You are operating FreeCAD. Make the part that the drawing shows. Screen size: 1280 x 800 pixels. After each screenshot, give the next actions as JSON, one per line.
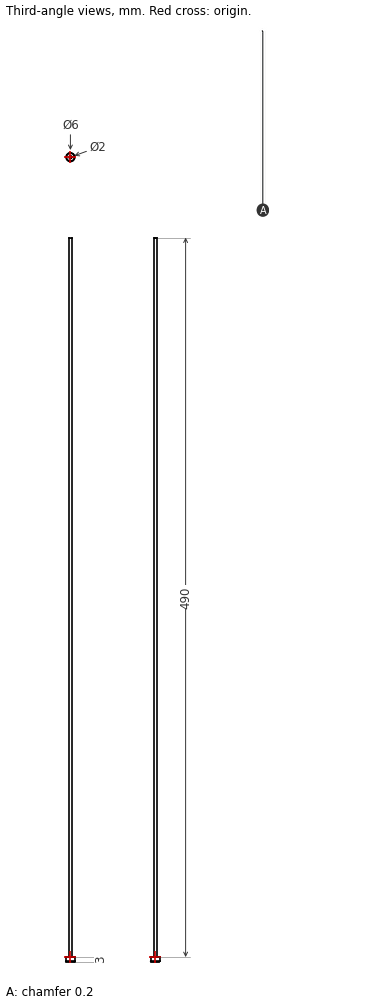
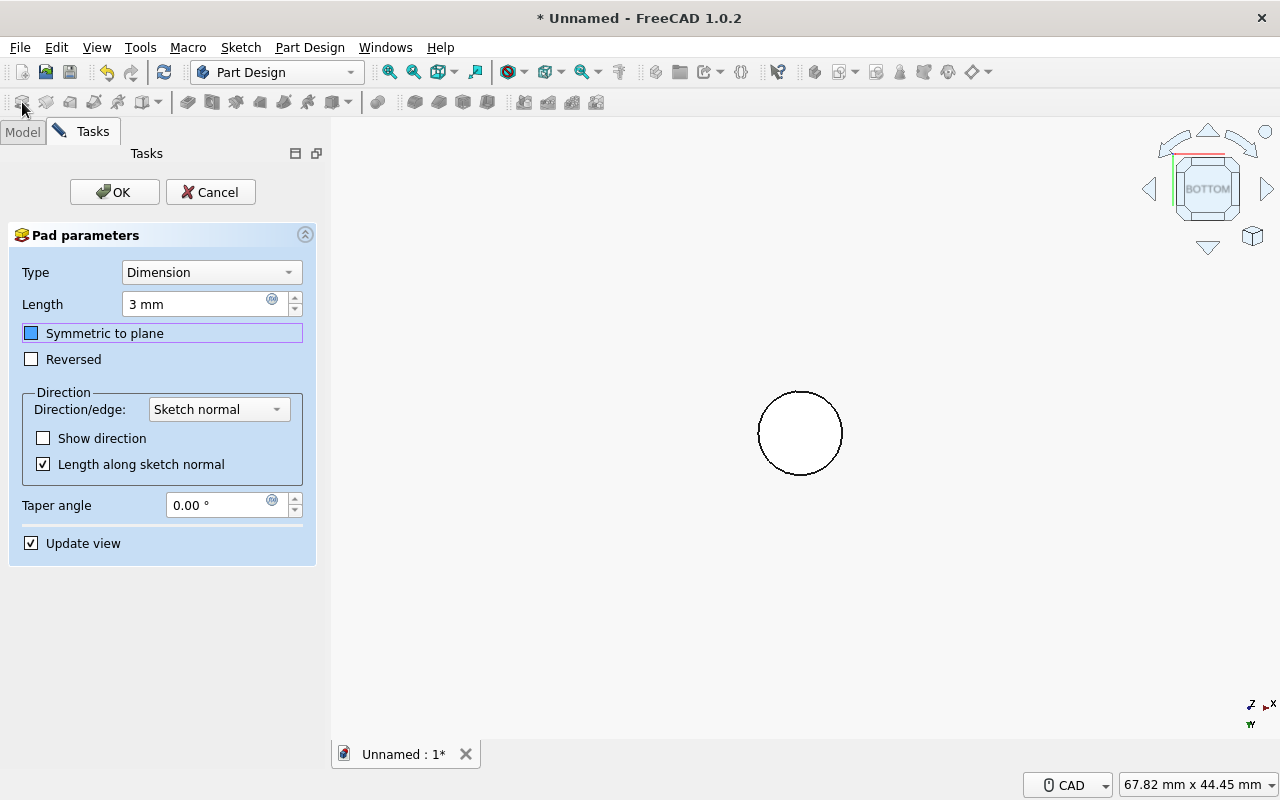
{"action": "left_click", "coordinate": [115, 192]}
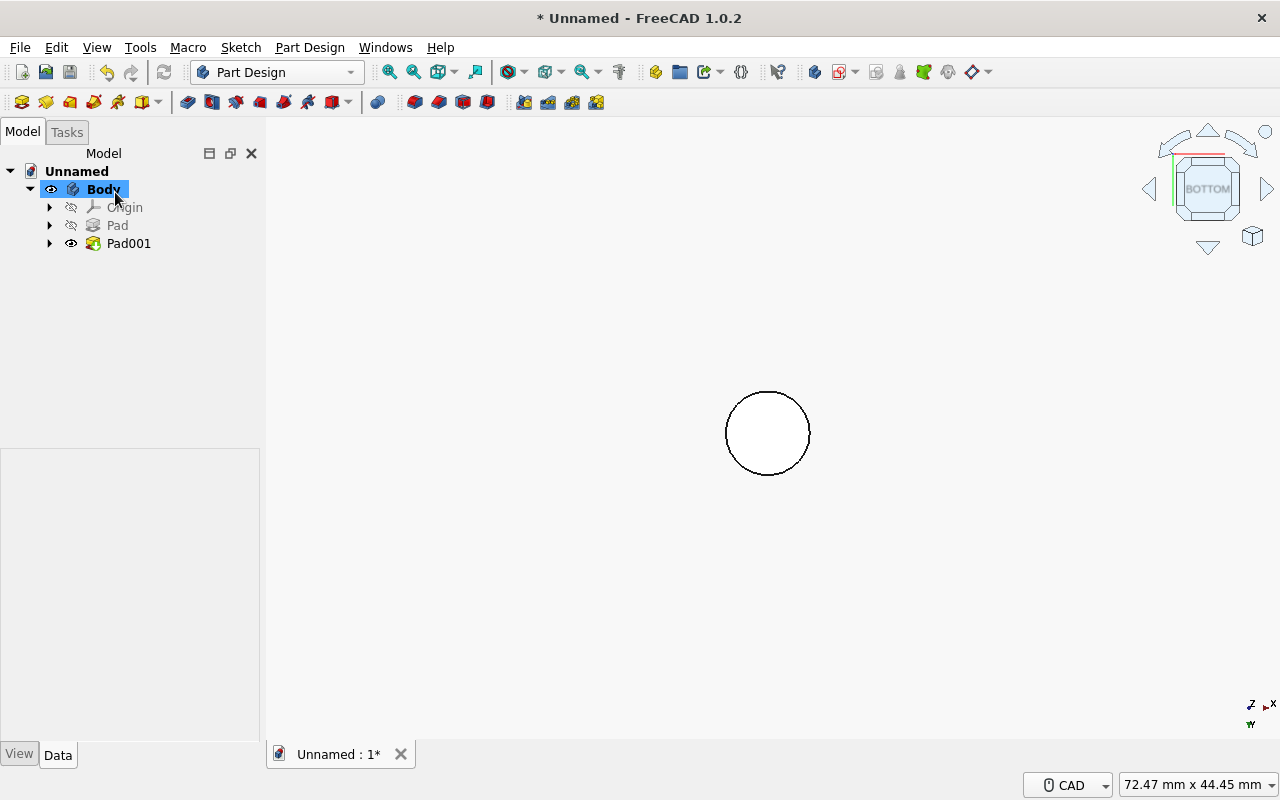
{"action": "key", "text": "v f"}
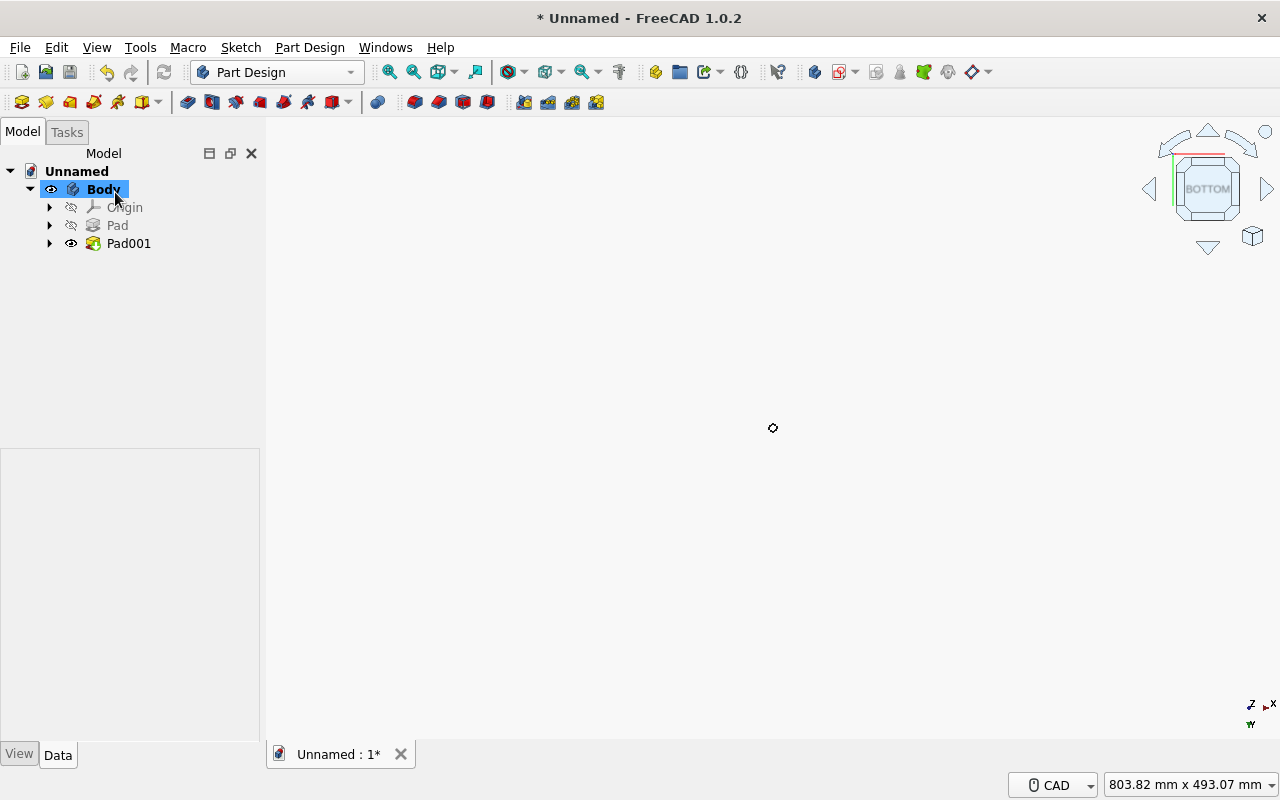
{"action": "left_click", "coordinate": [769, 427]}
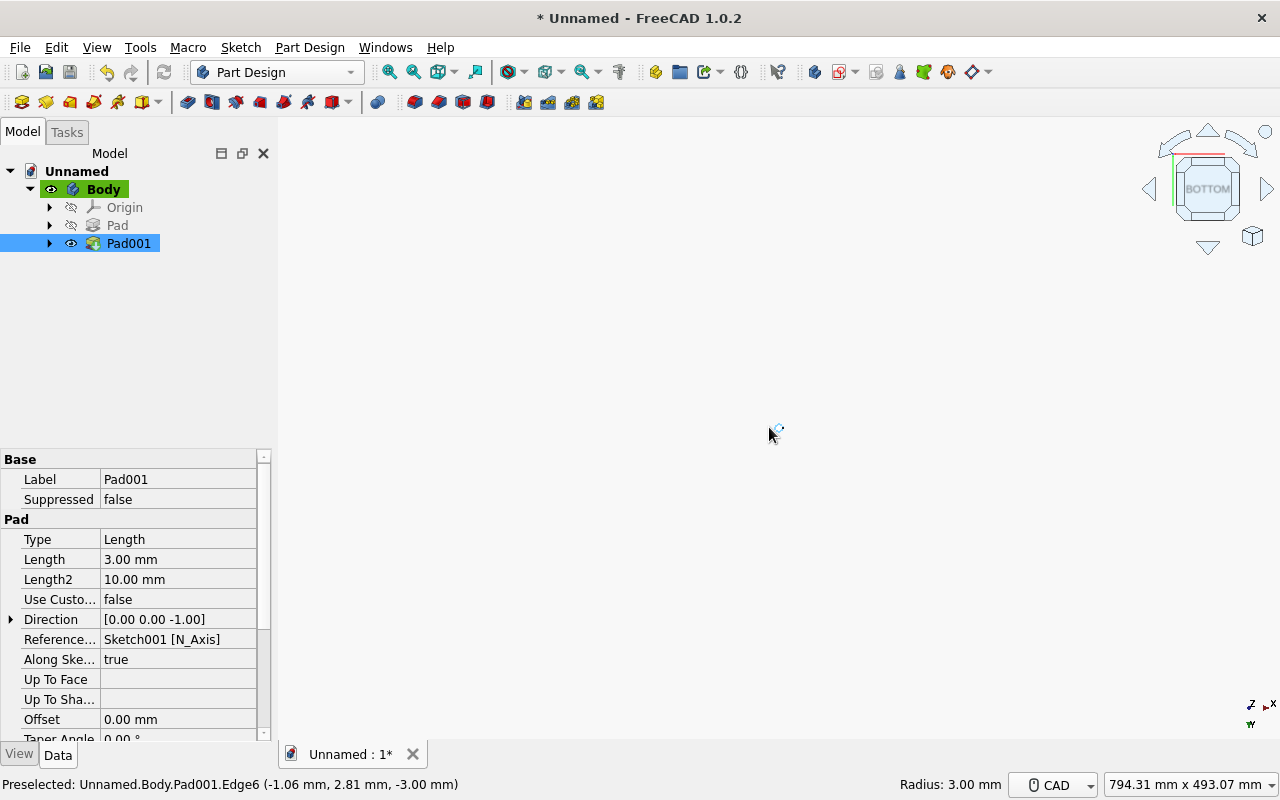
{"action": "key", "text": "0"}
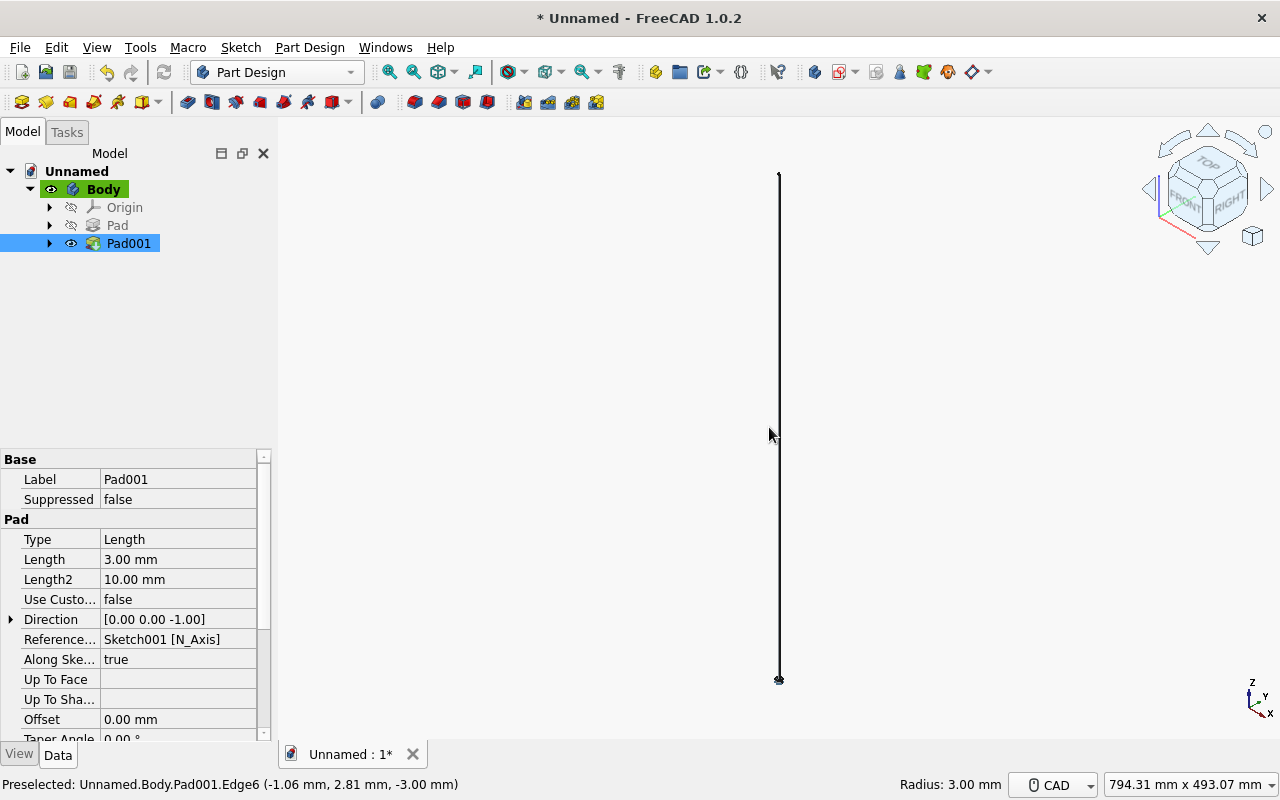
{"action": "left_click", "coordinate": [775, 677], "text": "ctrl"}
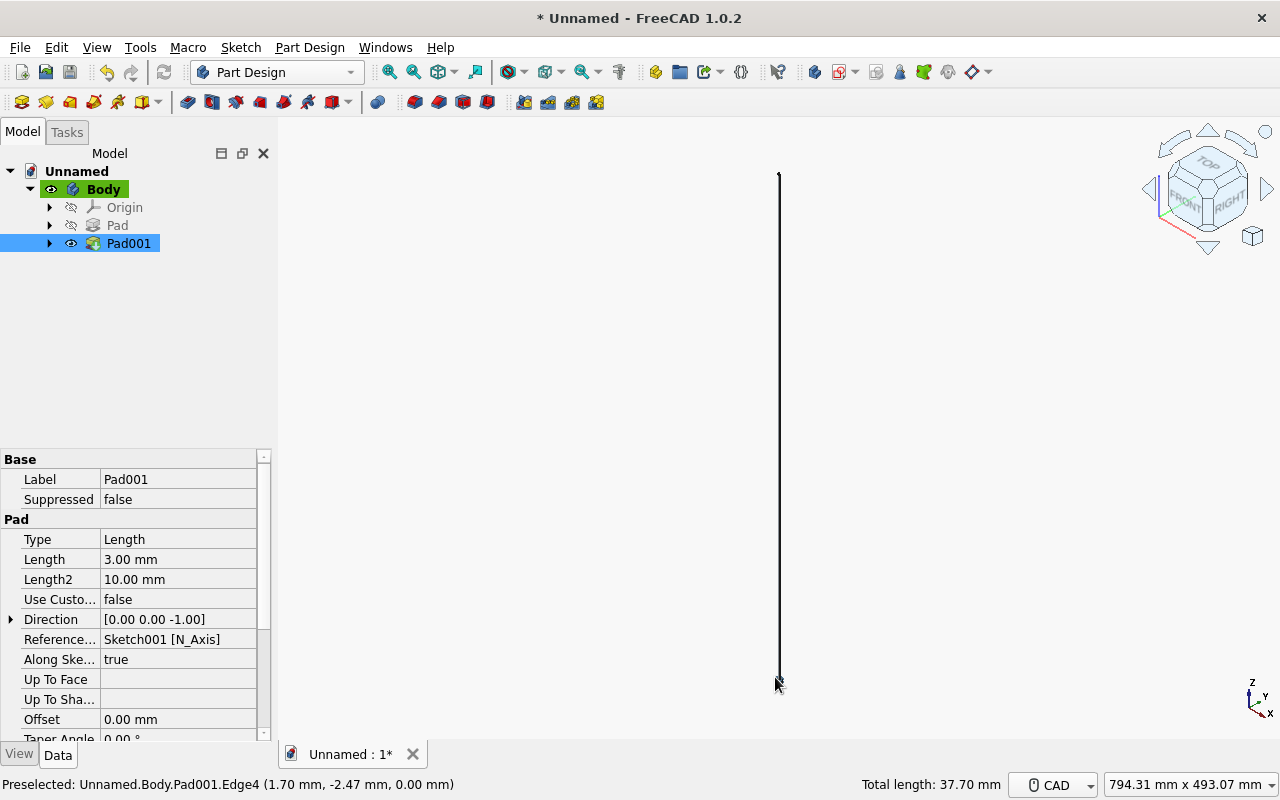
{"action": "left_click", "coordinate": [440, 102]}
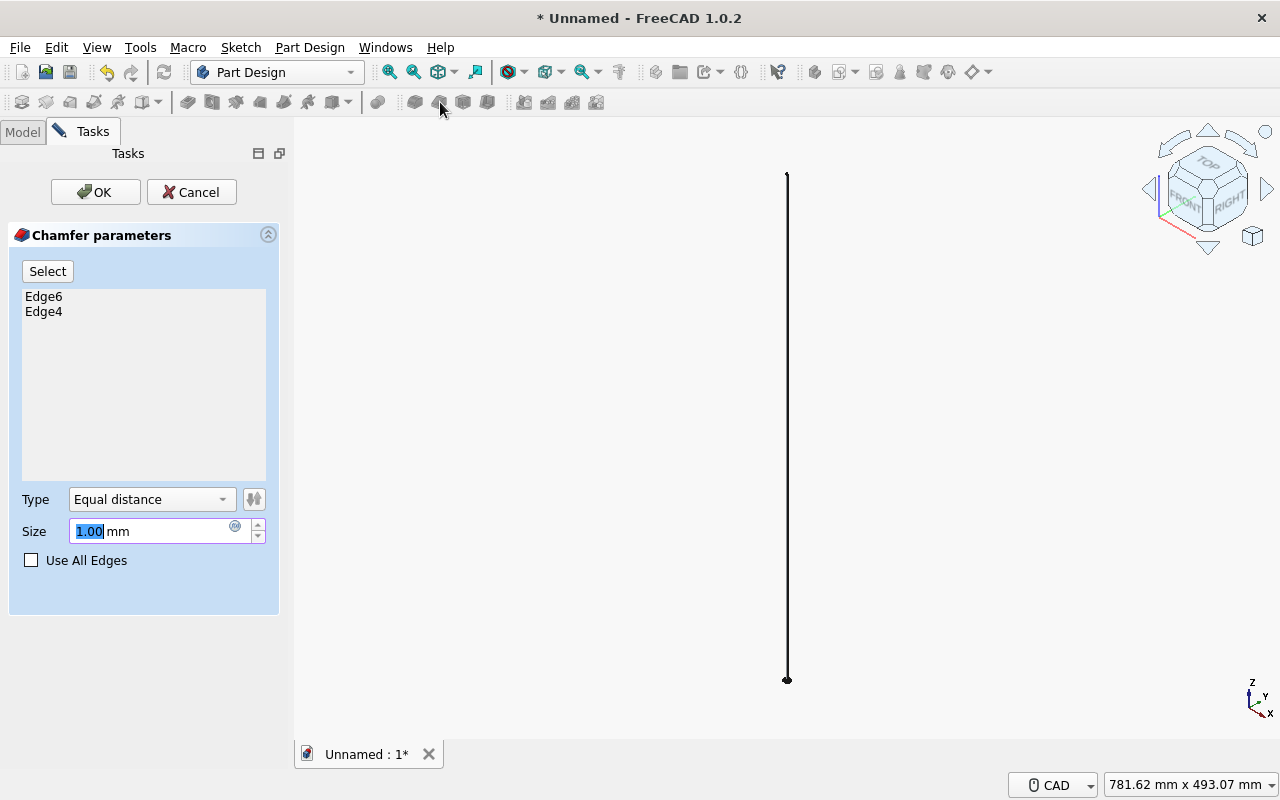
{"action": "type", "text": "0.2"}
{"action": "key", "text": "Tab"}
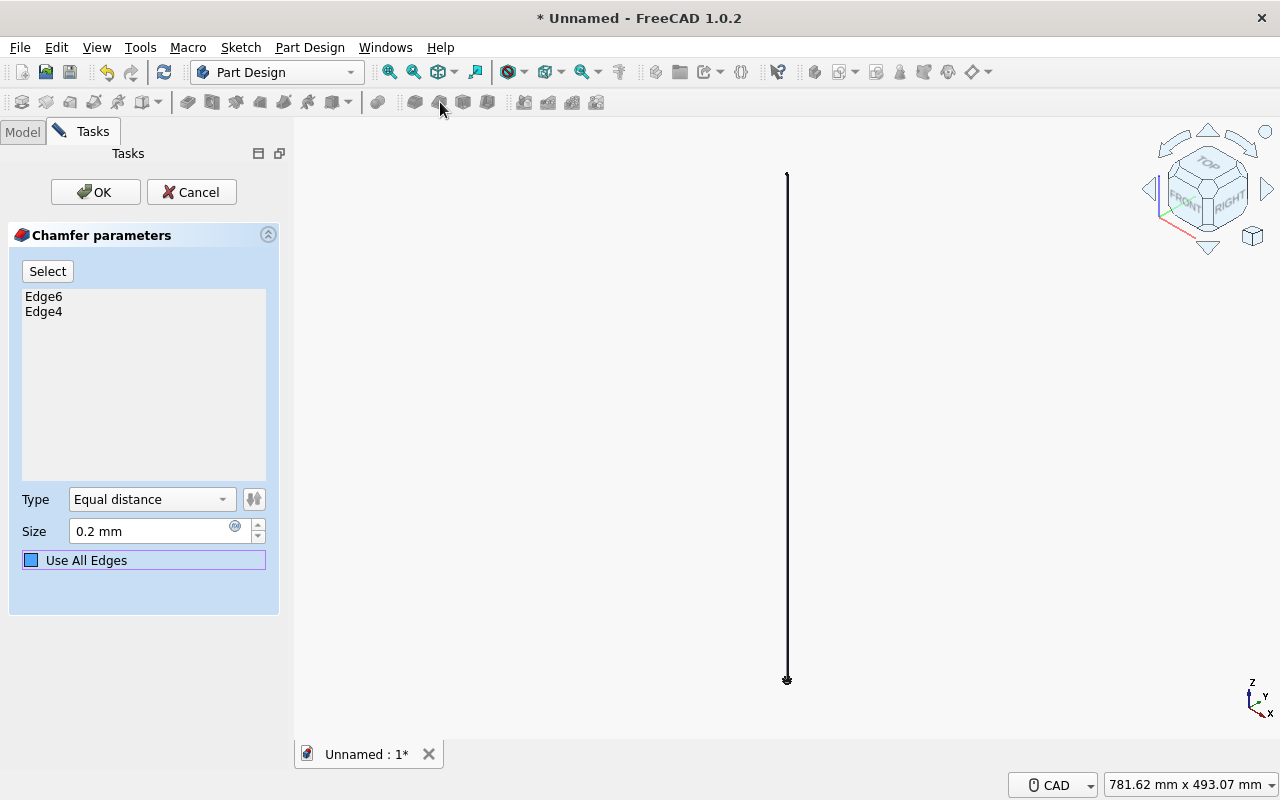
{"action": "left_click", "coordinate": [96, 192]}